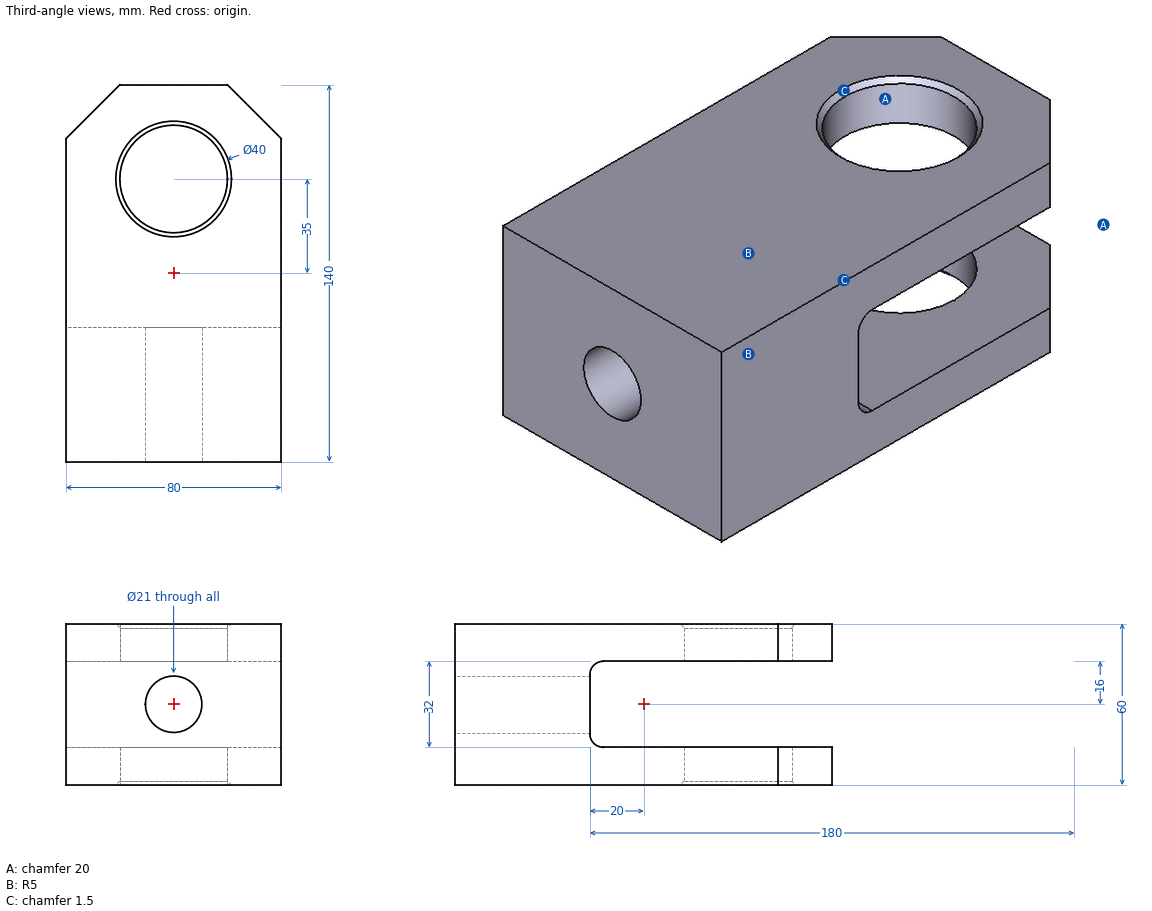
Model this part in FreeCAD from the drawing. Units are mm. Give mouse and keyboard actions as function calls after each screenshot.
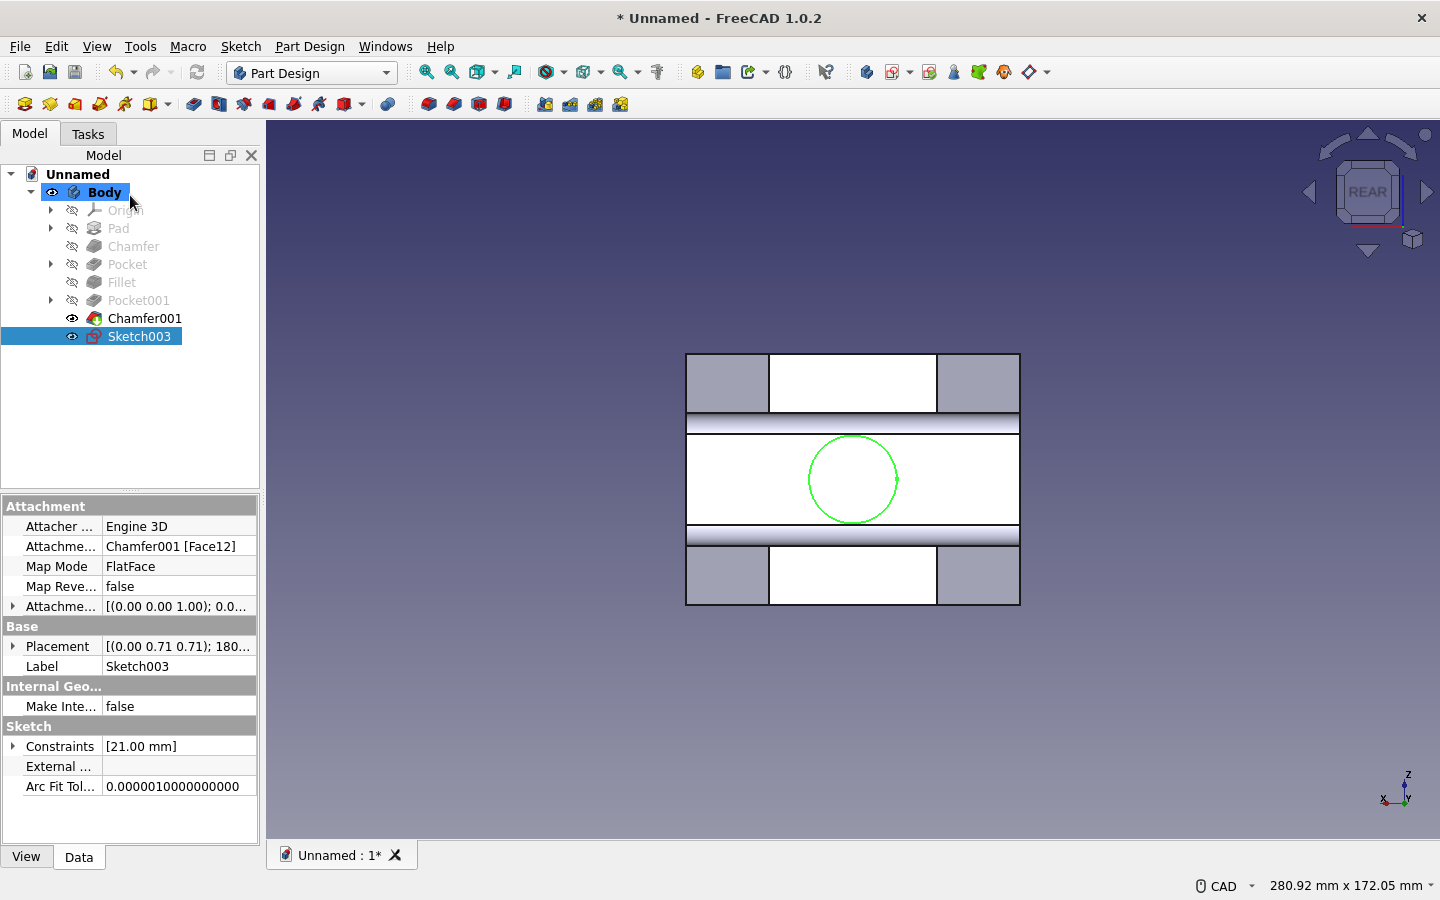
click(219, 104)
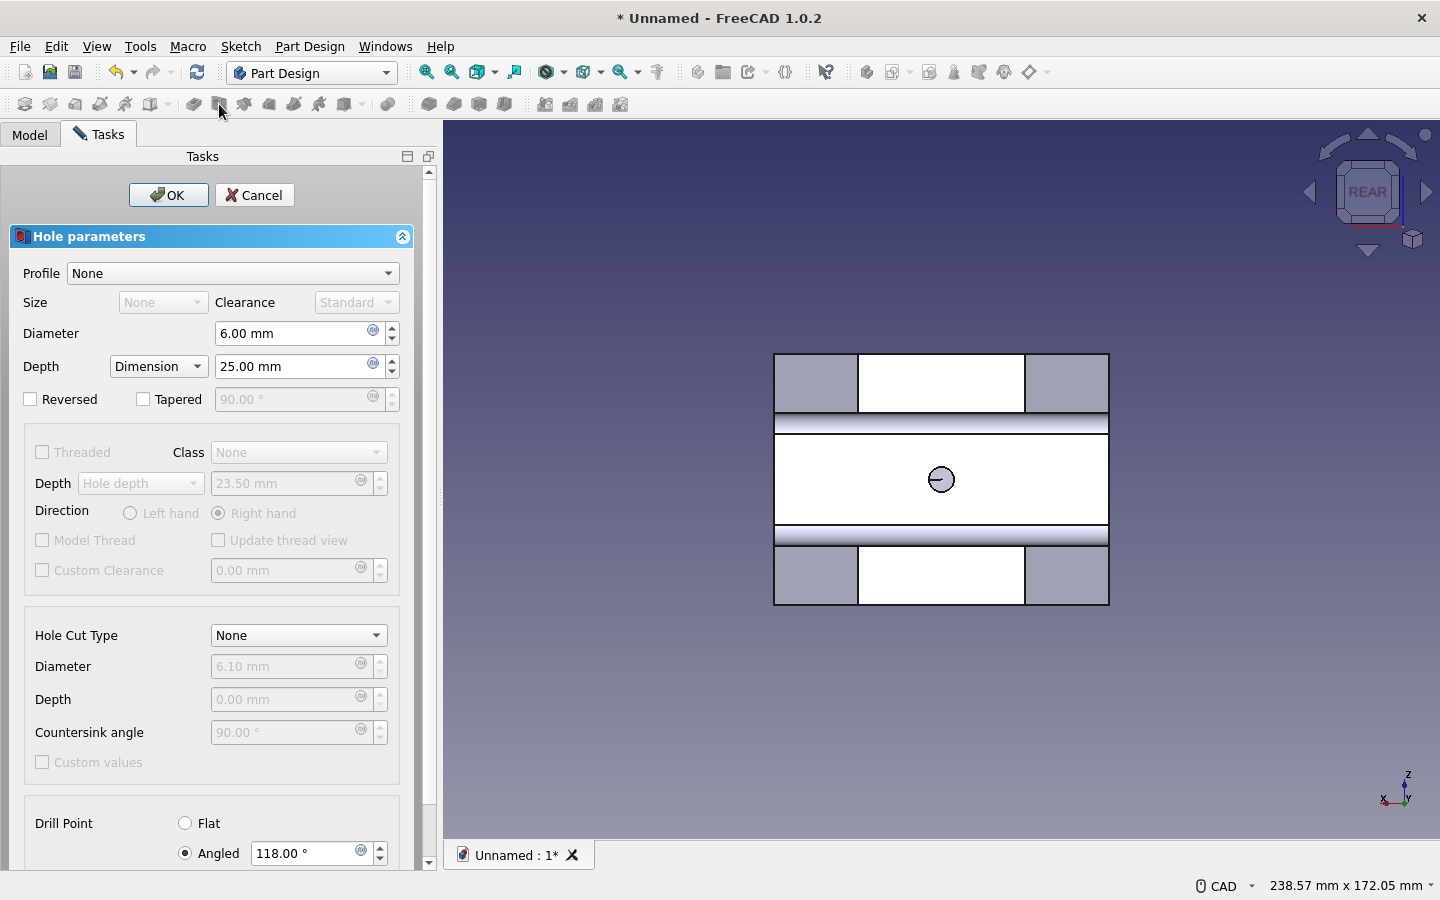
triple_click(300, 334)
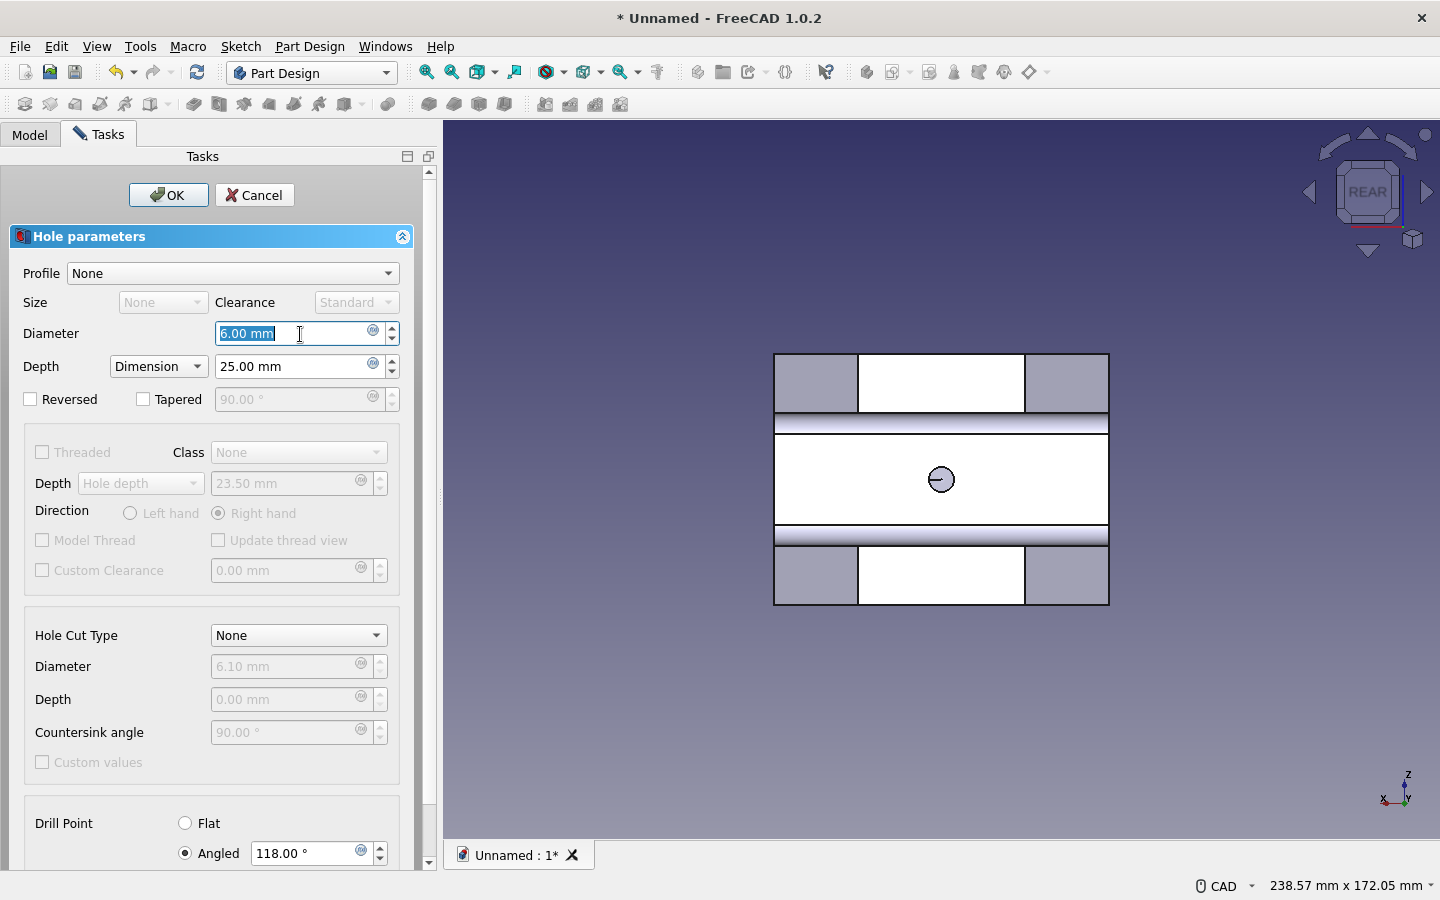
text(21)
key(Tab)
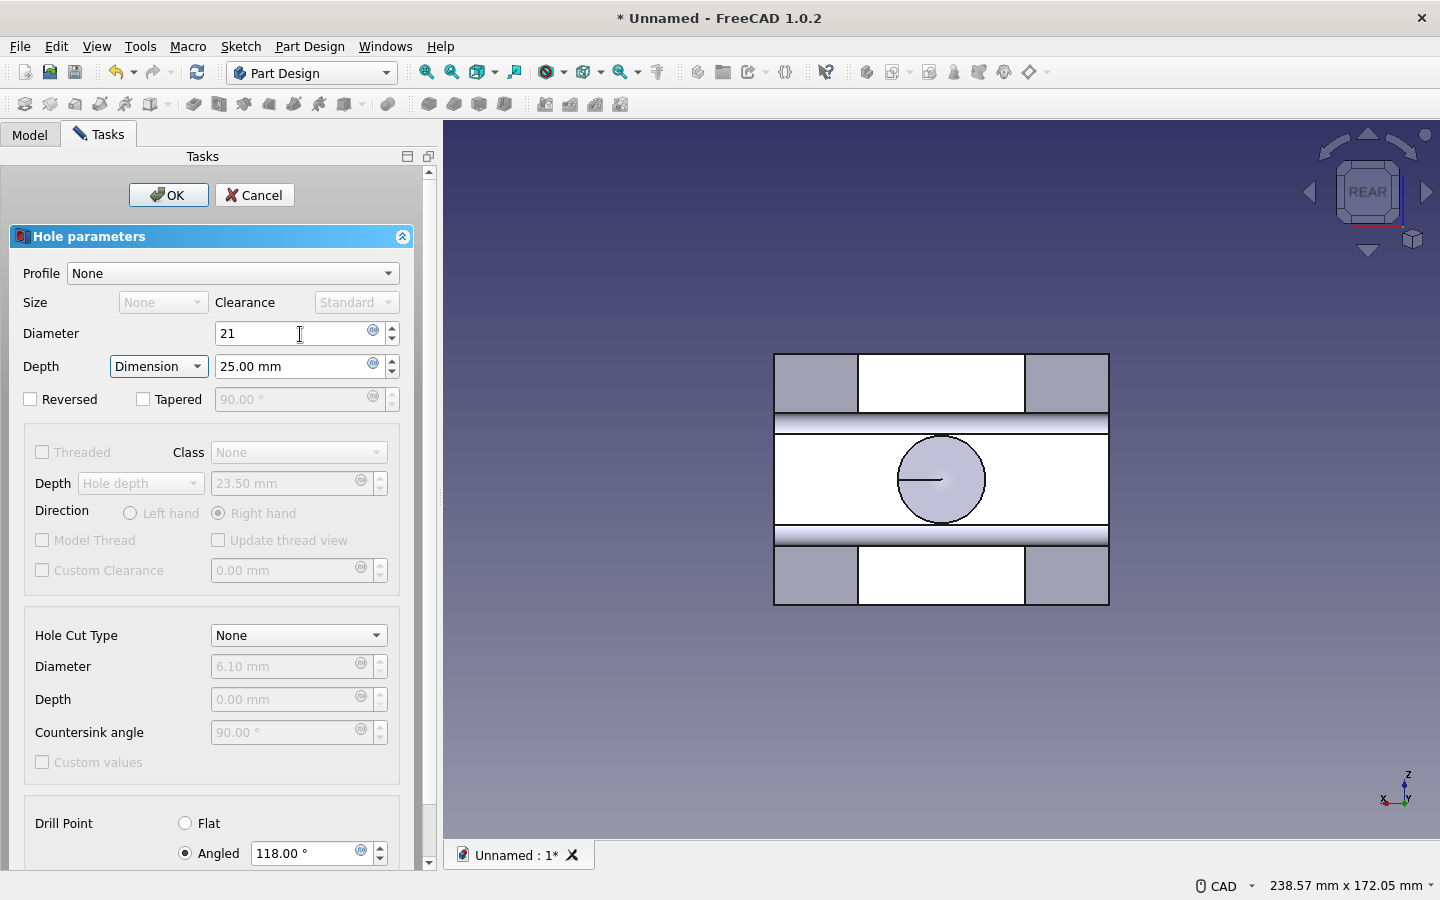
click(160, 366)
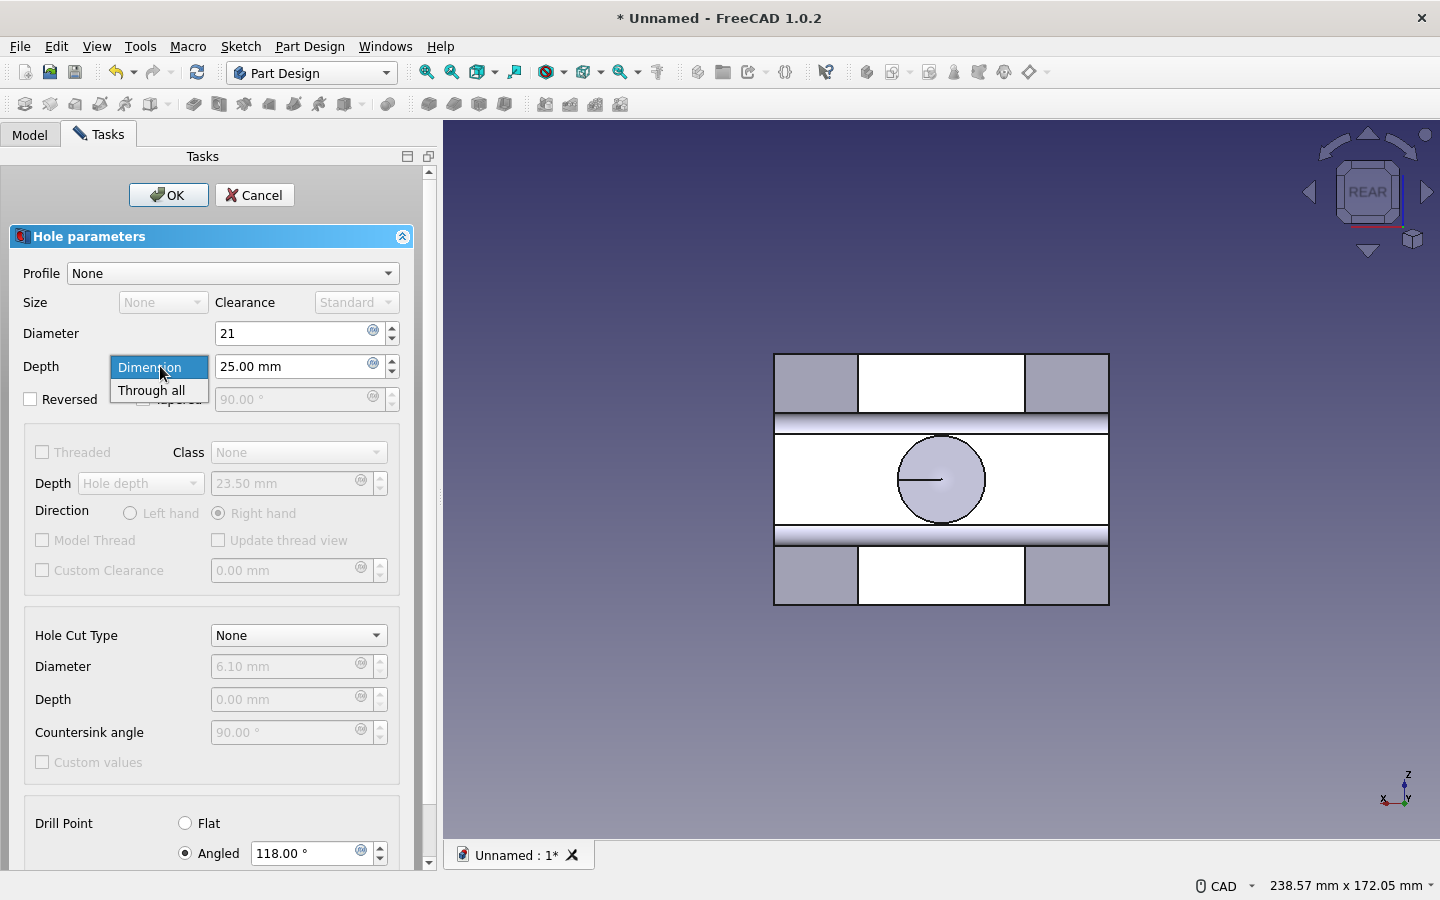
click(158, 390)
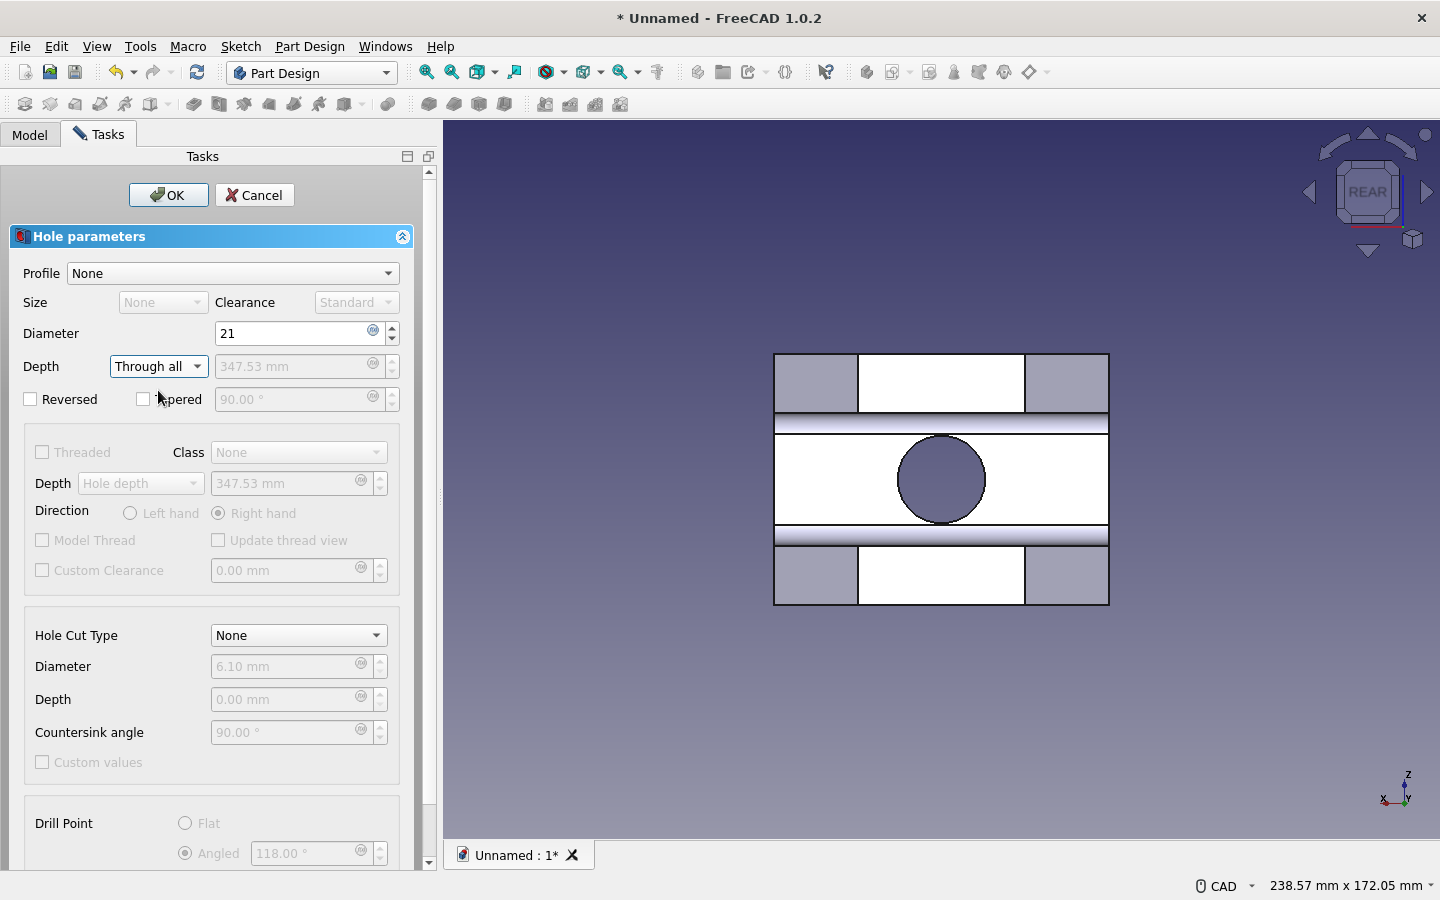
click(169, 195)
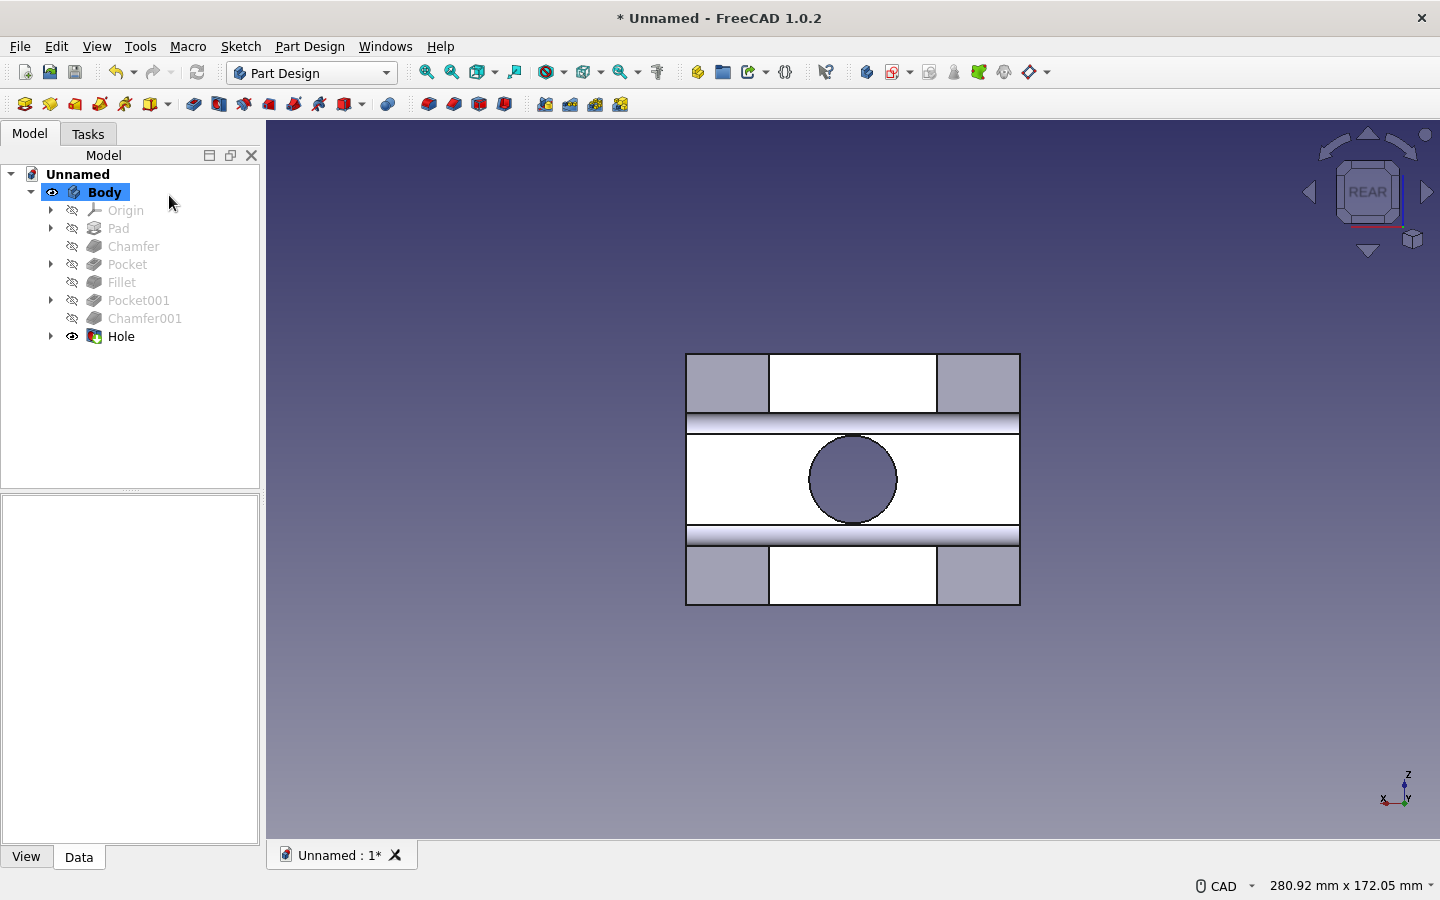
key(0)